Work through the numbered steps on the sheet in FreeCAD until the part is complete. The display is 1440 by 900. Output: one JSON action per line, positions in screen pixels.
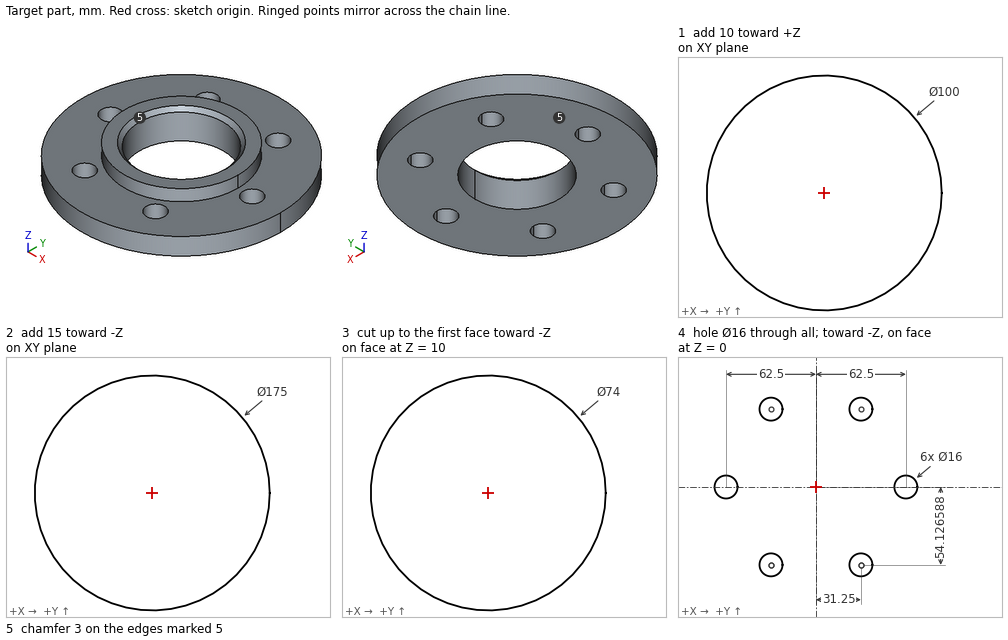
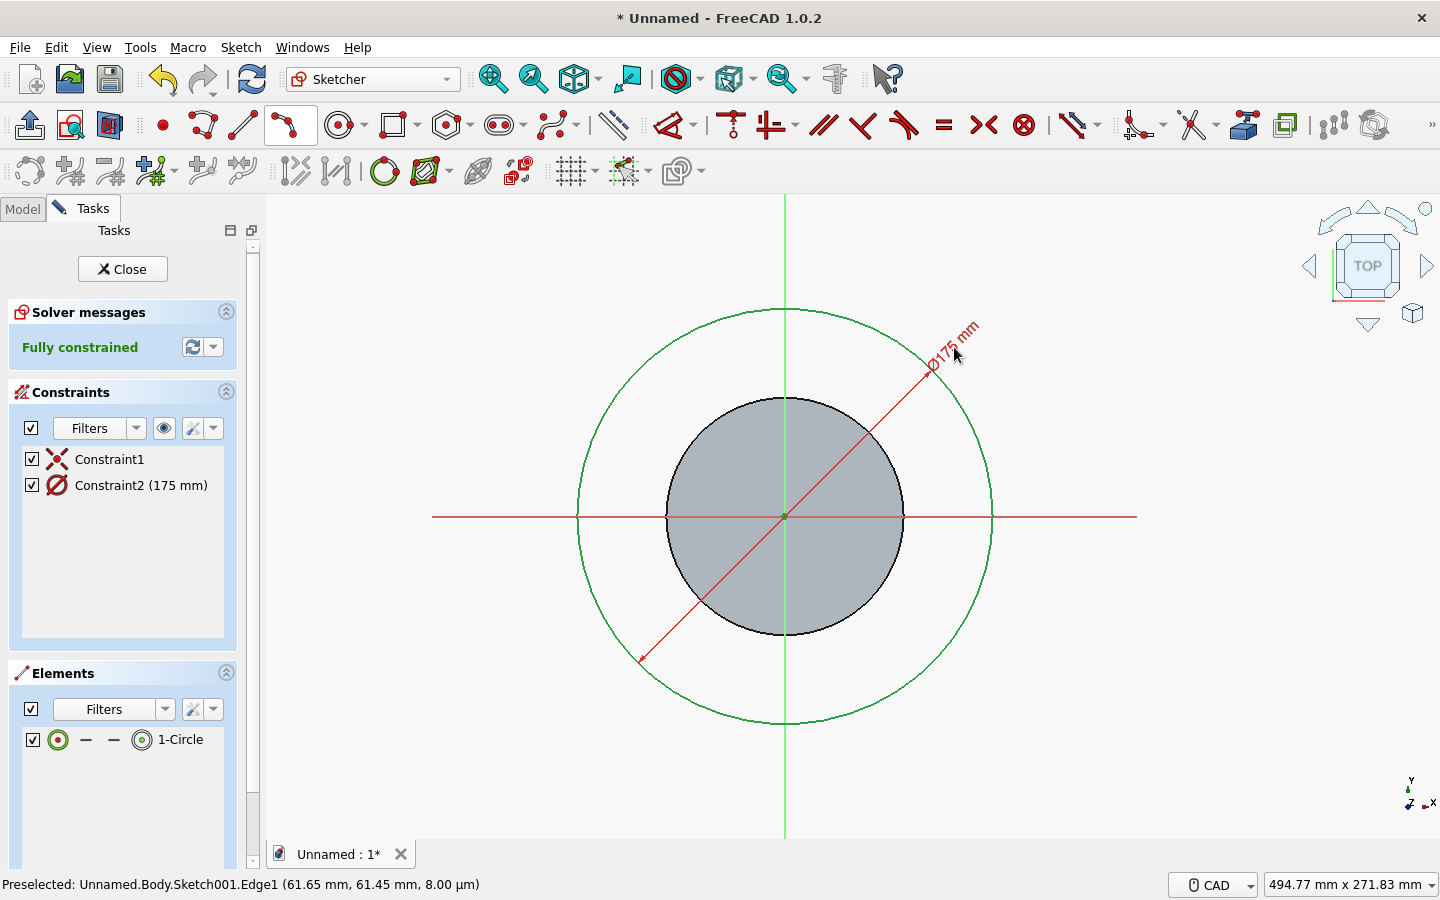
{"action": "left_click", "coordinate": [123, 269]}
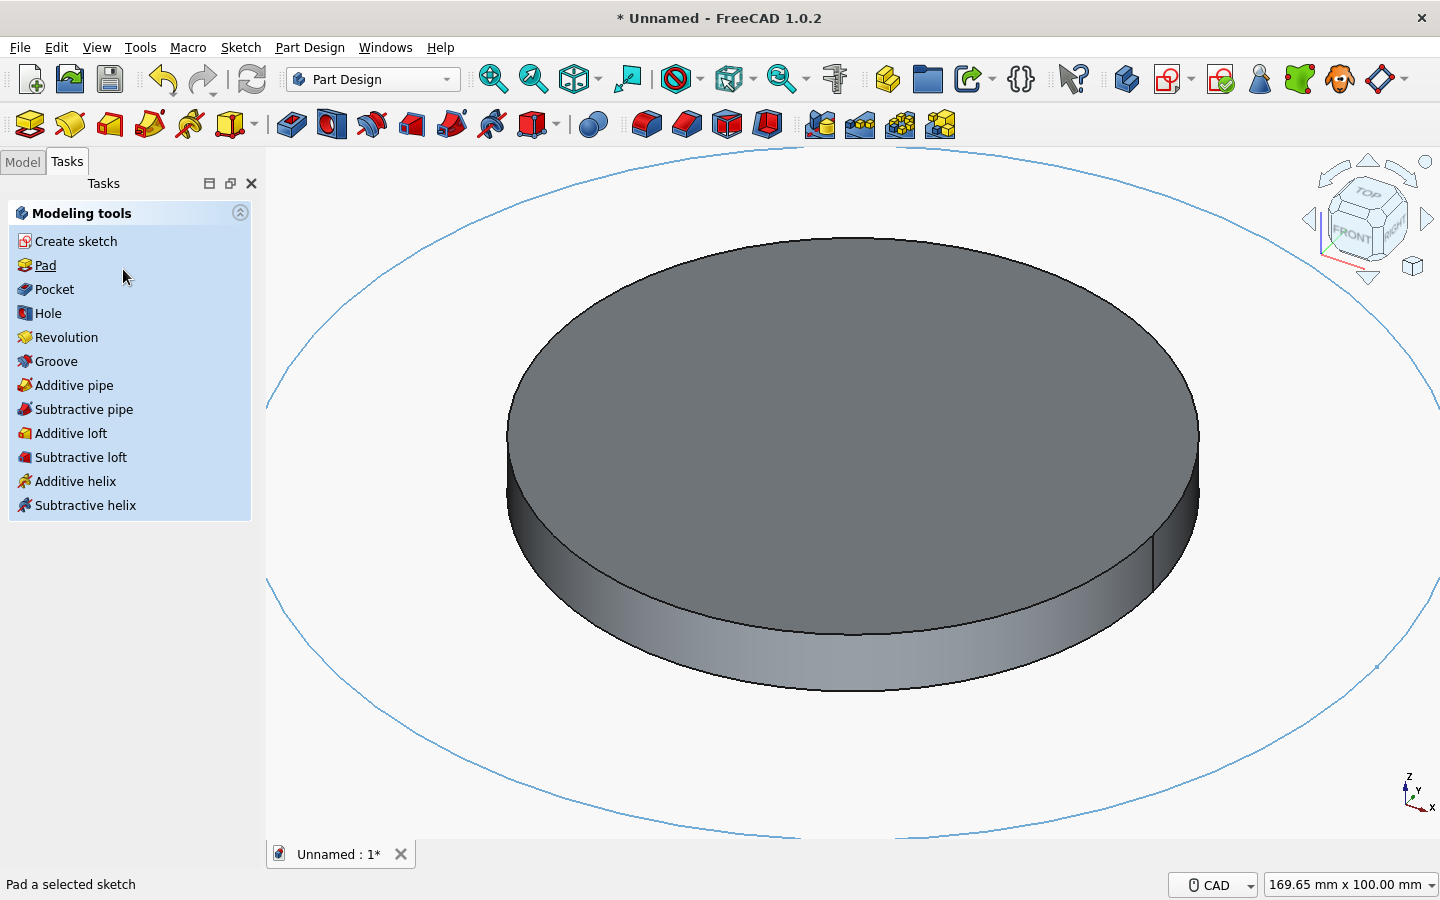
{"action": "left_click", "coordinate": [30, 124]}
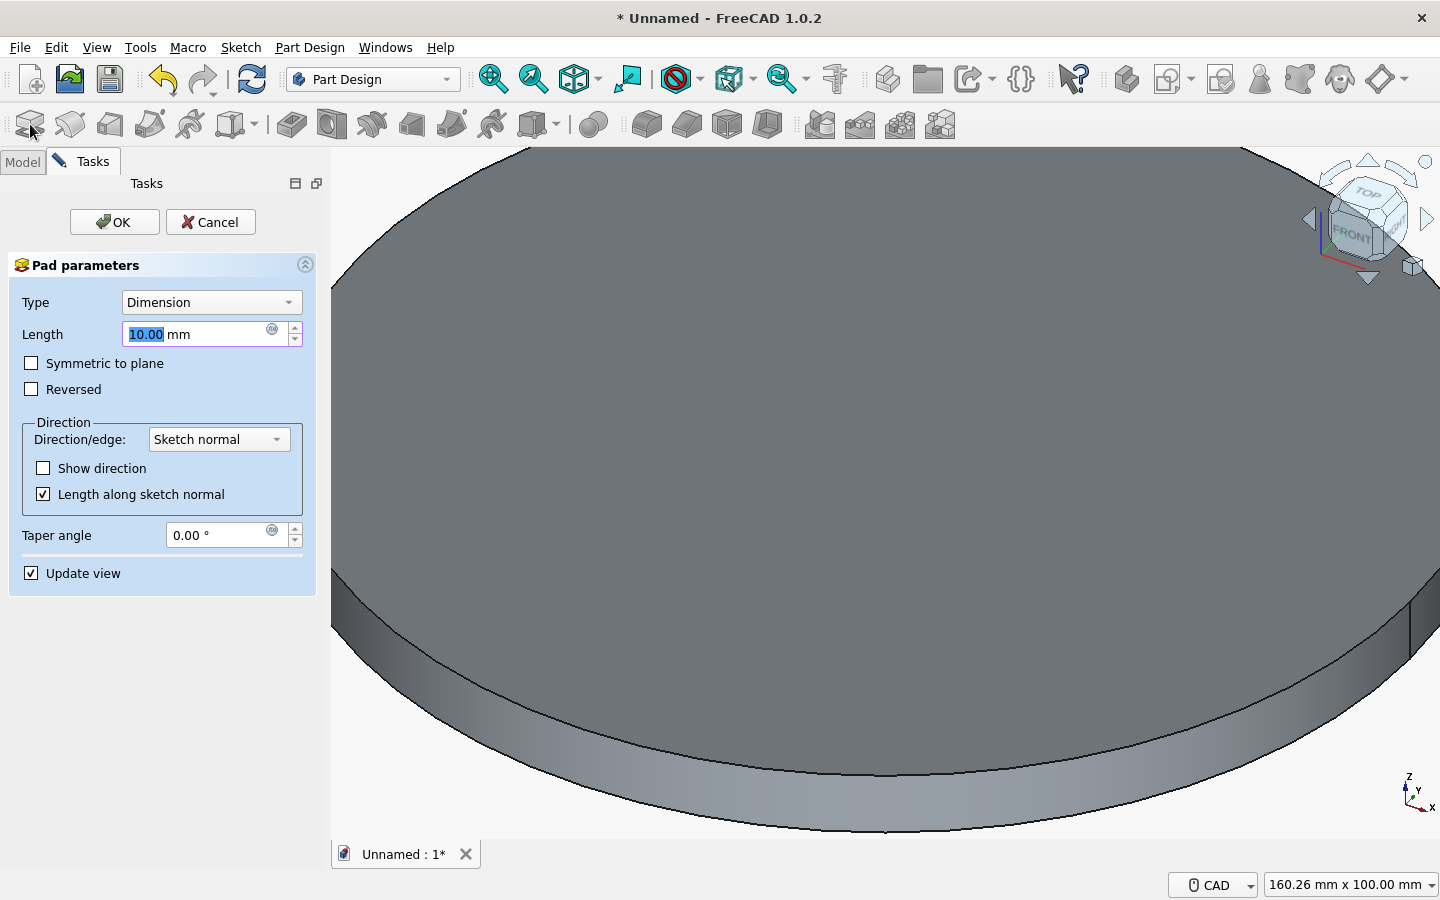
{"action": "type", "text": "15"}
{"action": "key", "text": "Tab"}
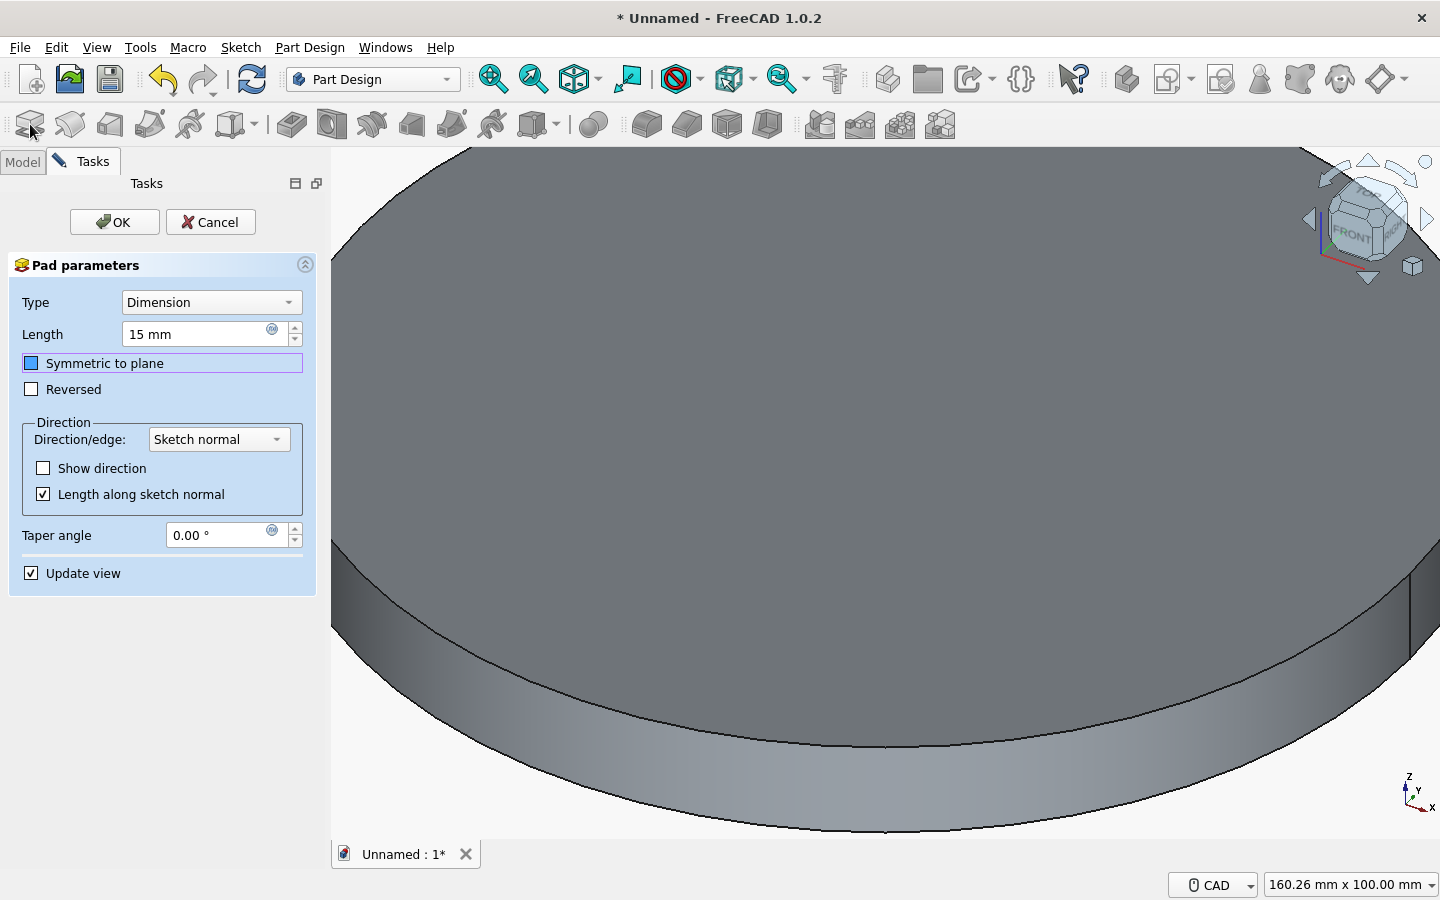
{"action": "left_click", "coordinate": [30, 389]}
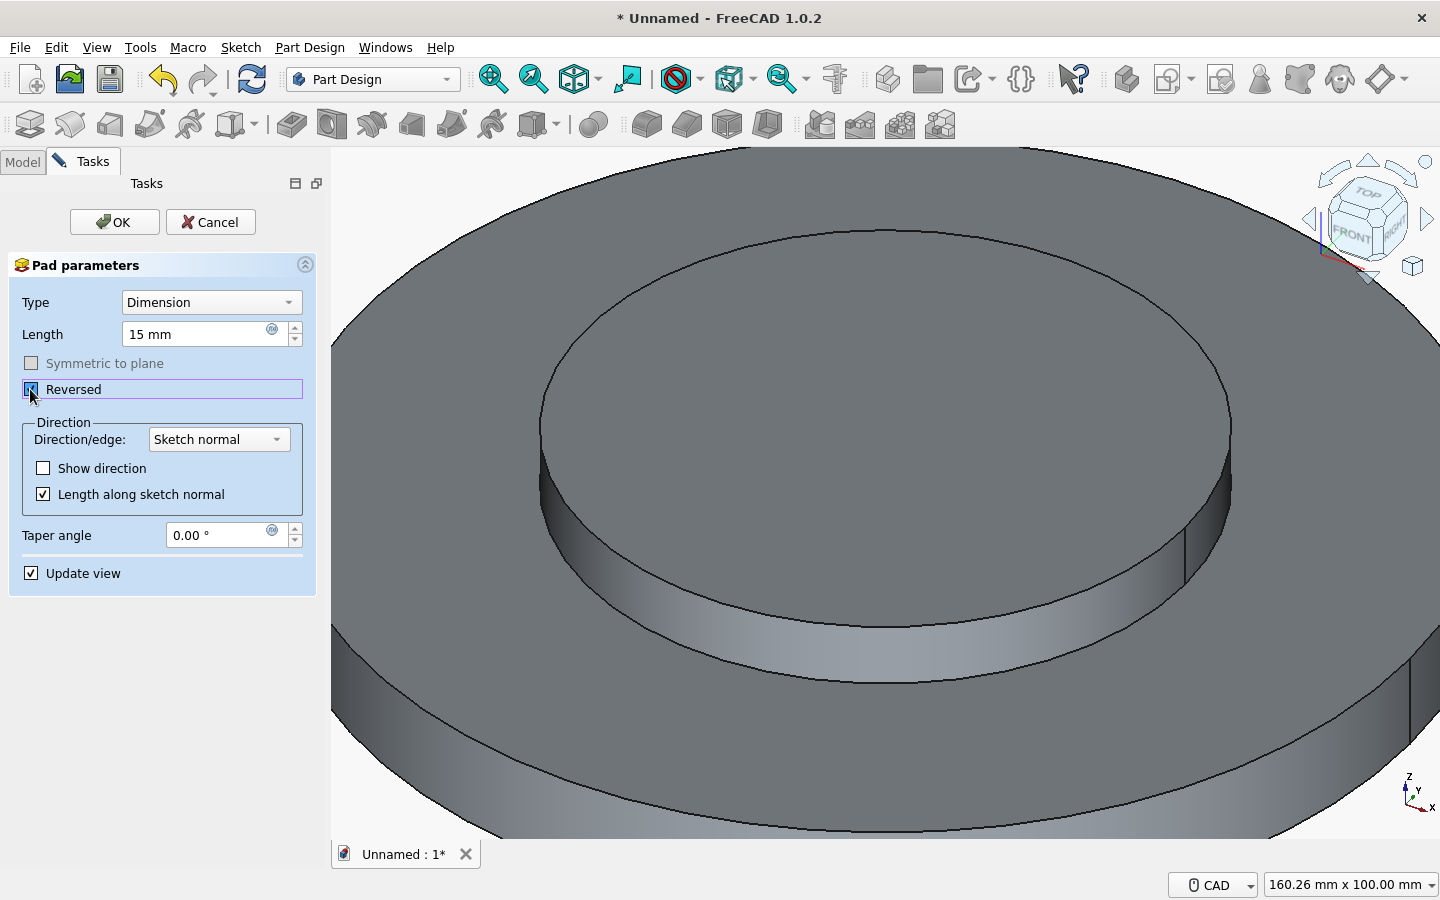
{"action": "left_click", "coordinate": [115, 222]}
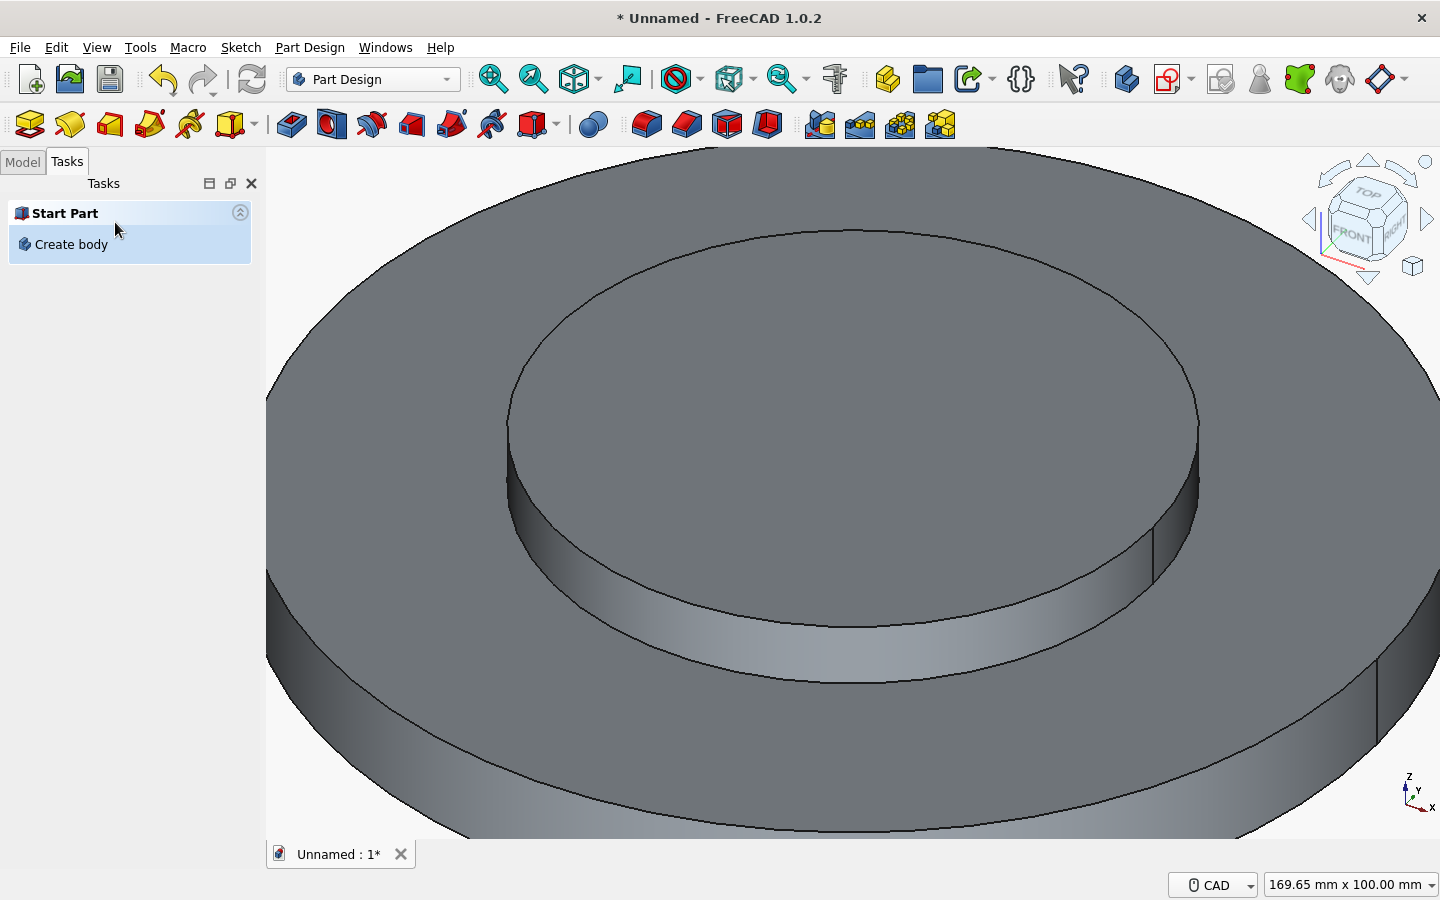
{"action": "left_click", "coordinate": [494, 80]}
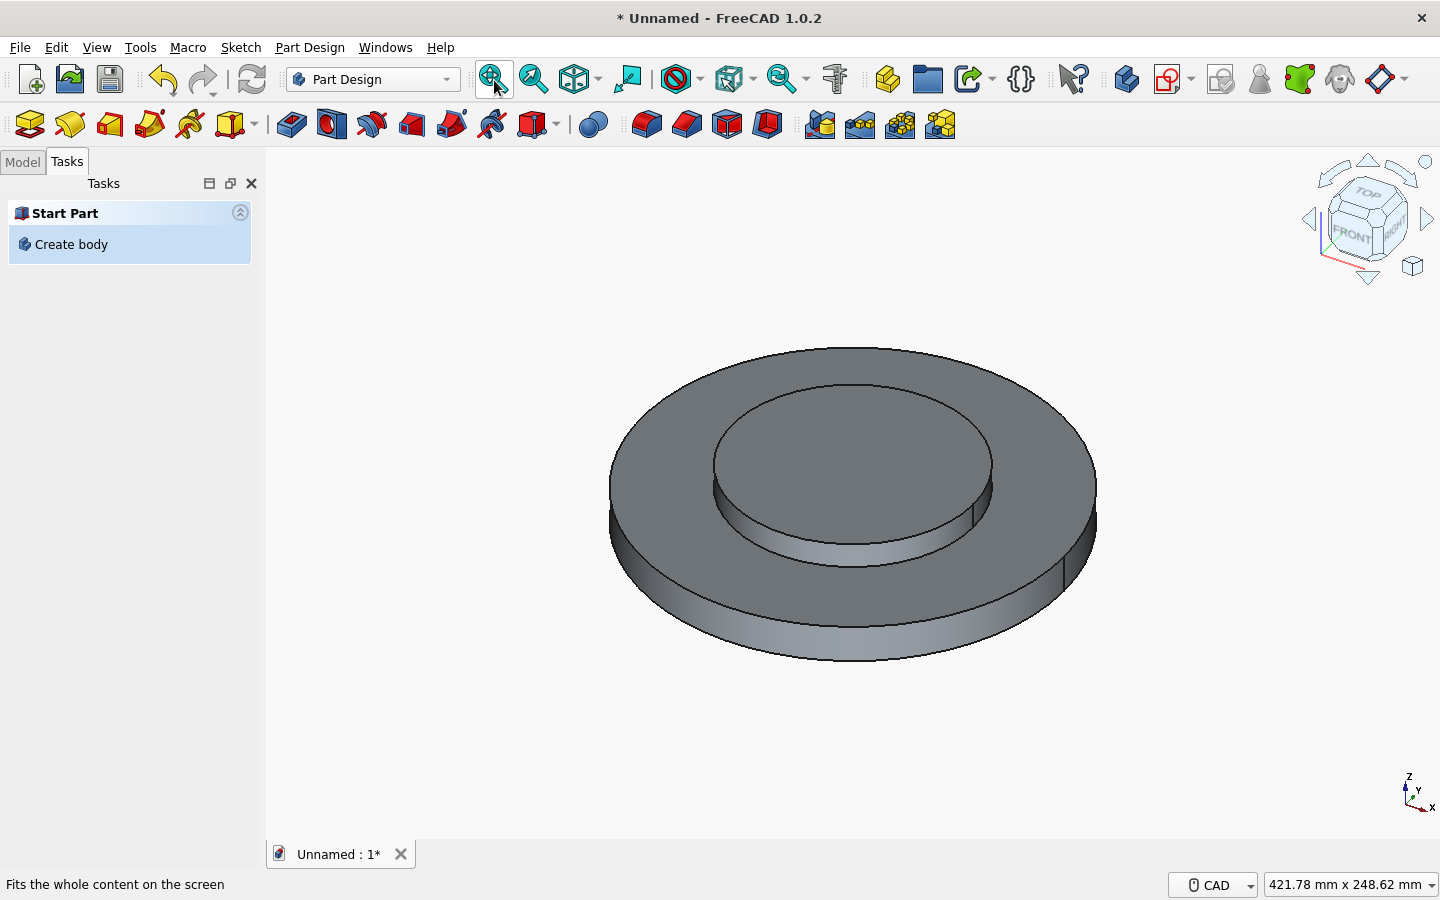
{"action": "left_click", "coordinate": [853, 463]}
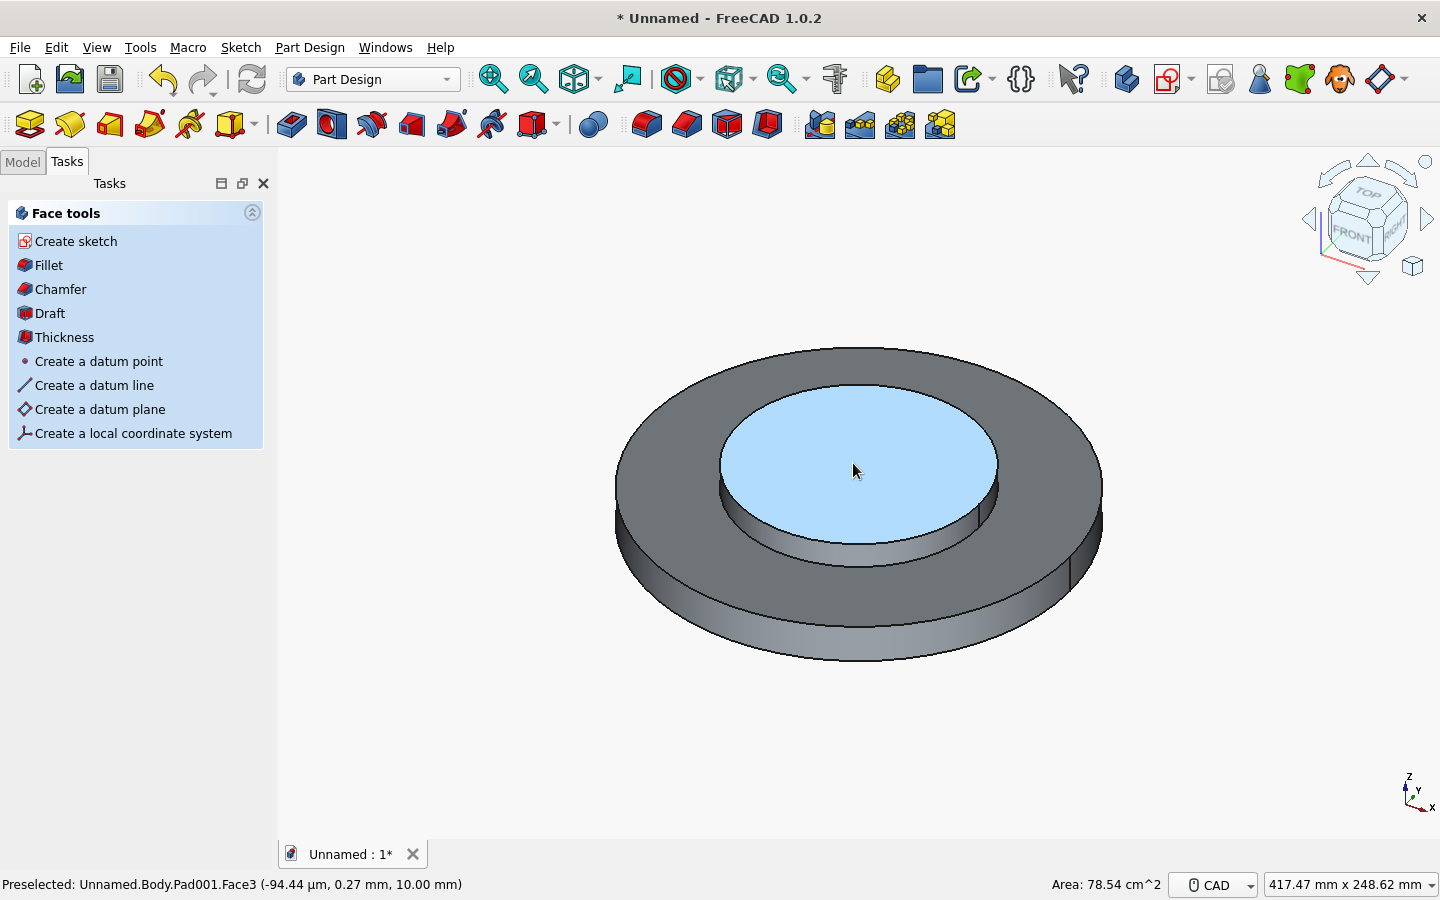
{"action": "left_click", "coordinate": [1168, 80]}